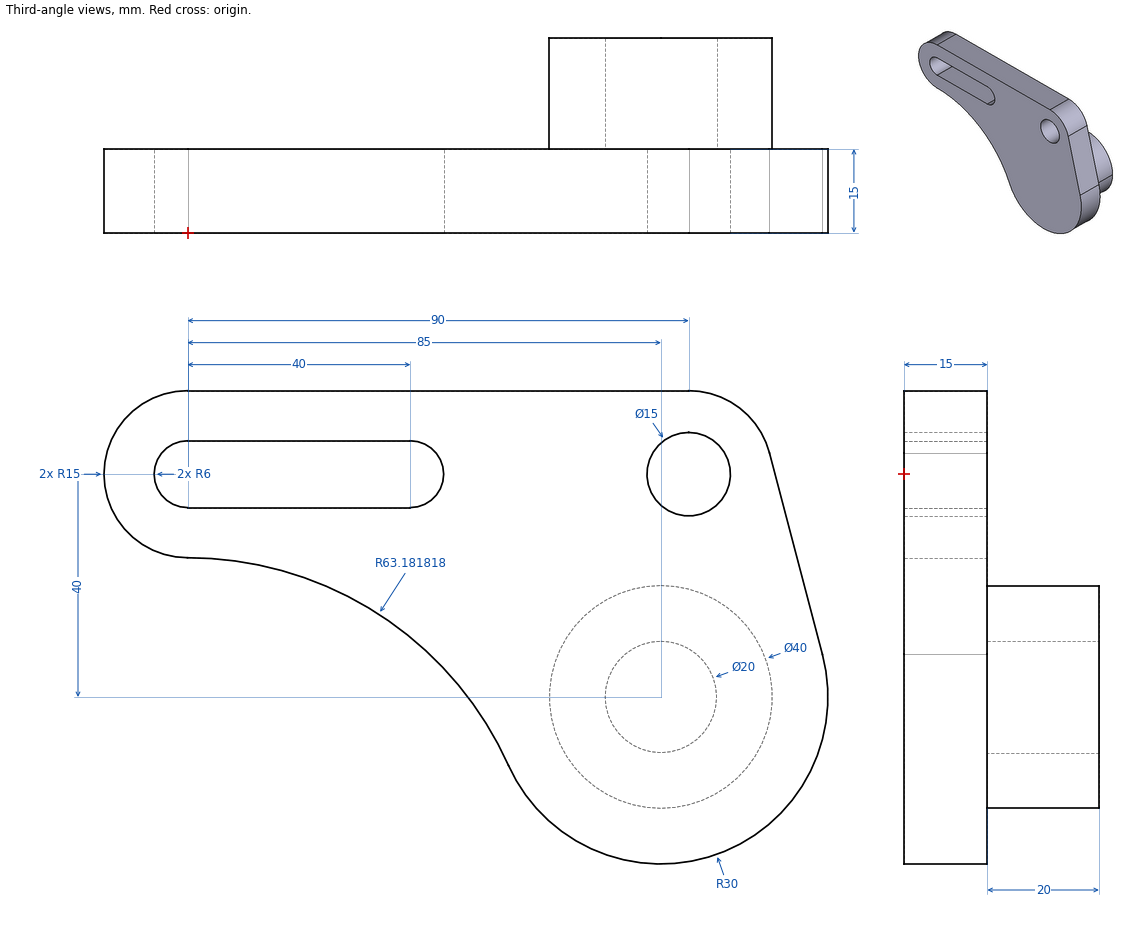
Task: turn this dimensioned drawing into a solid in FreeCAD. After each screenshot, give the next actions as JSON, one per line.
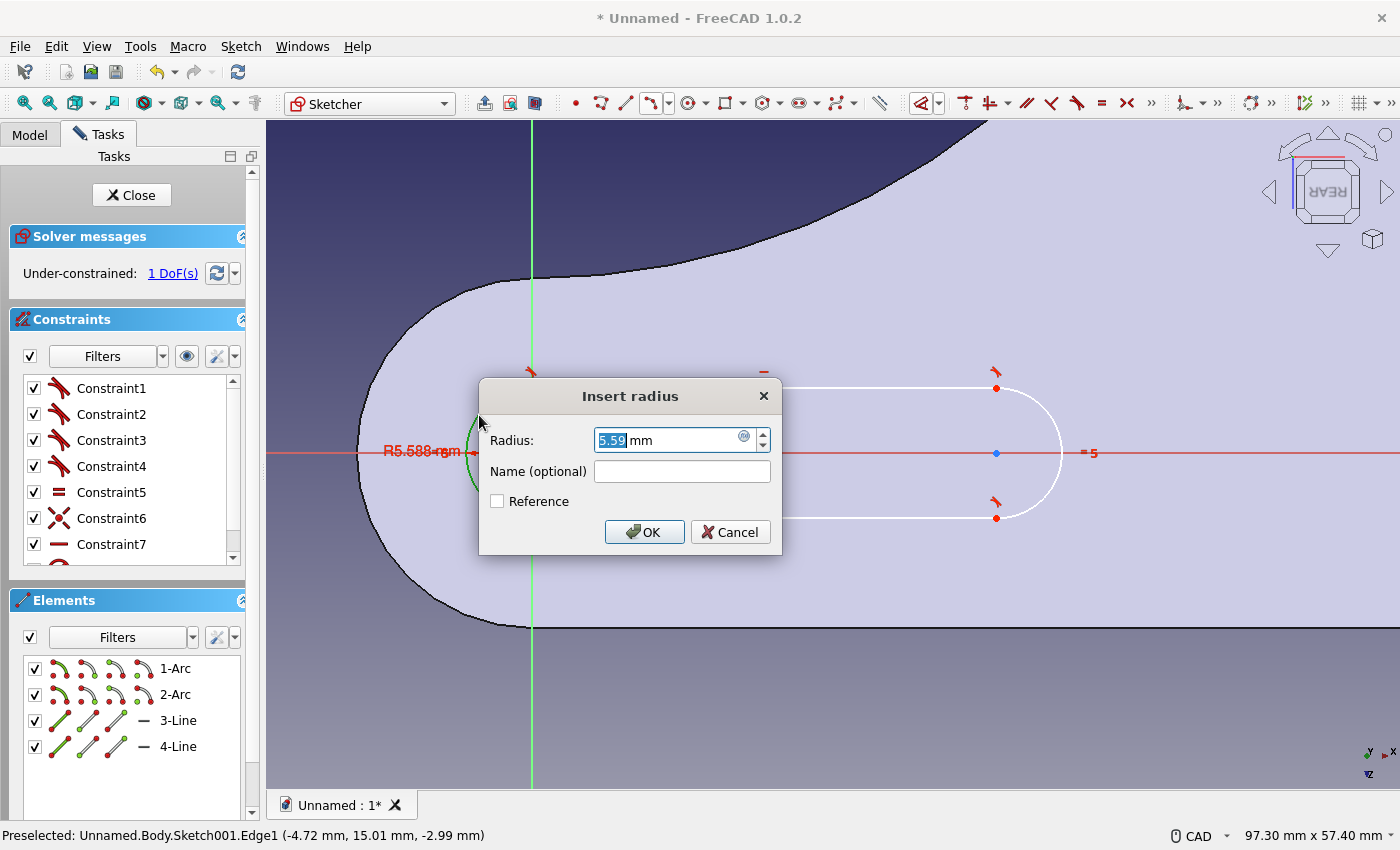
{"action": "type", "text": "6"}
{"action": "key", "text": "Return"}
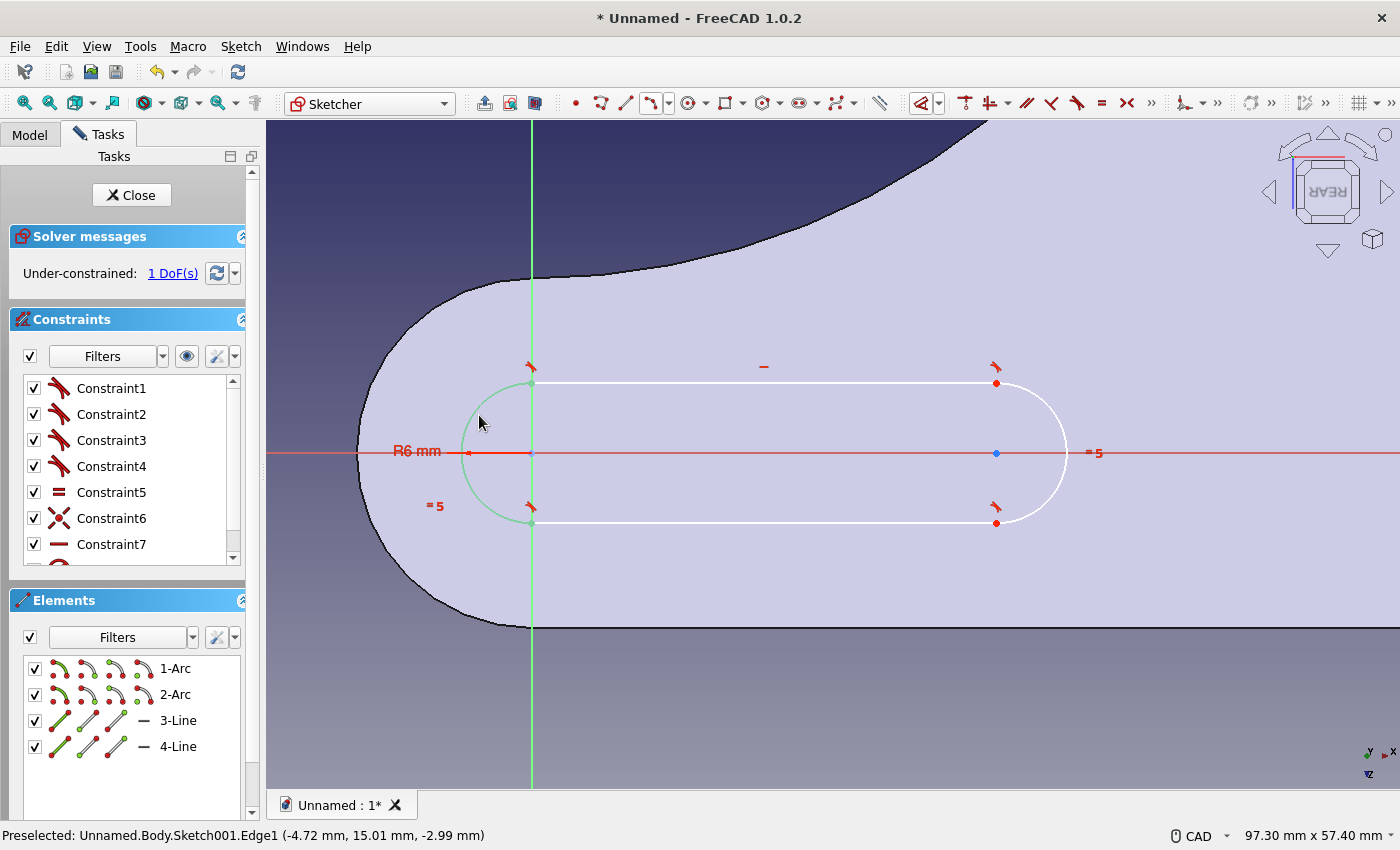
{"action": "left_click", "coordinate": [671, 383]}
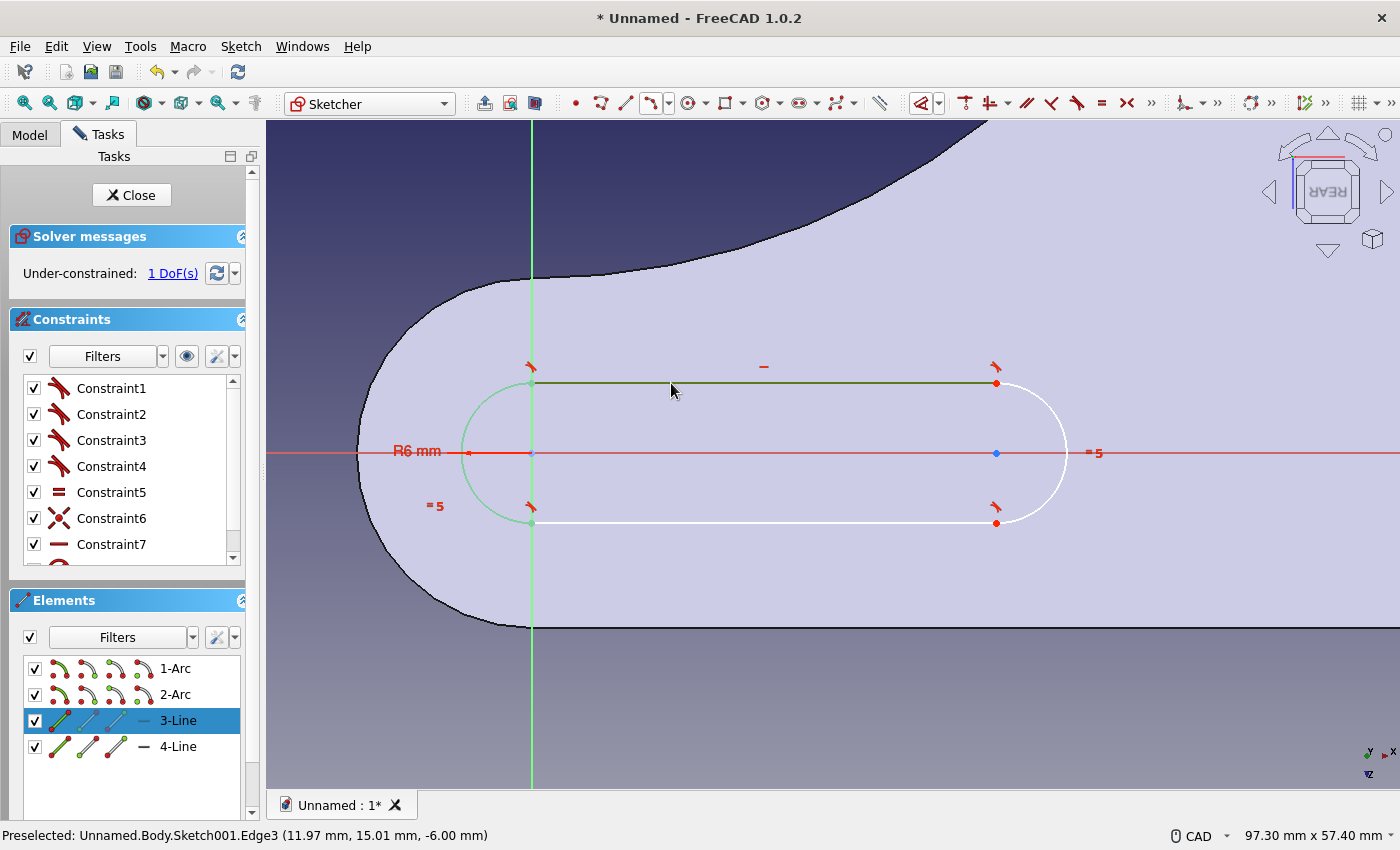
{"action": "left_click", "coordinate": [938, 104]}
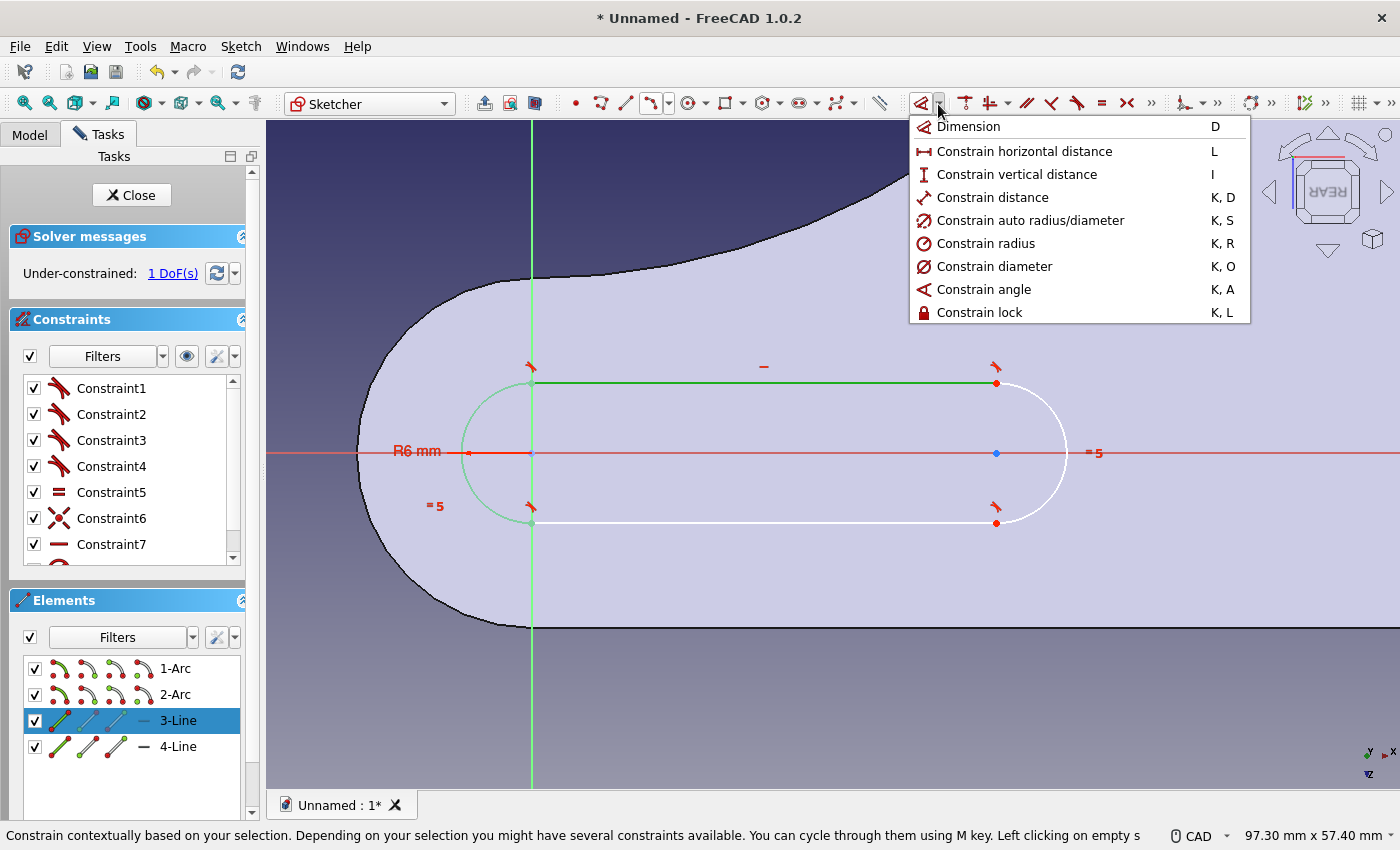
{"action": "left_click", "coordinate": [1080, 152]}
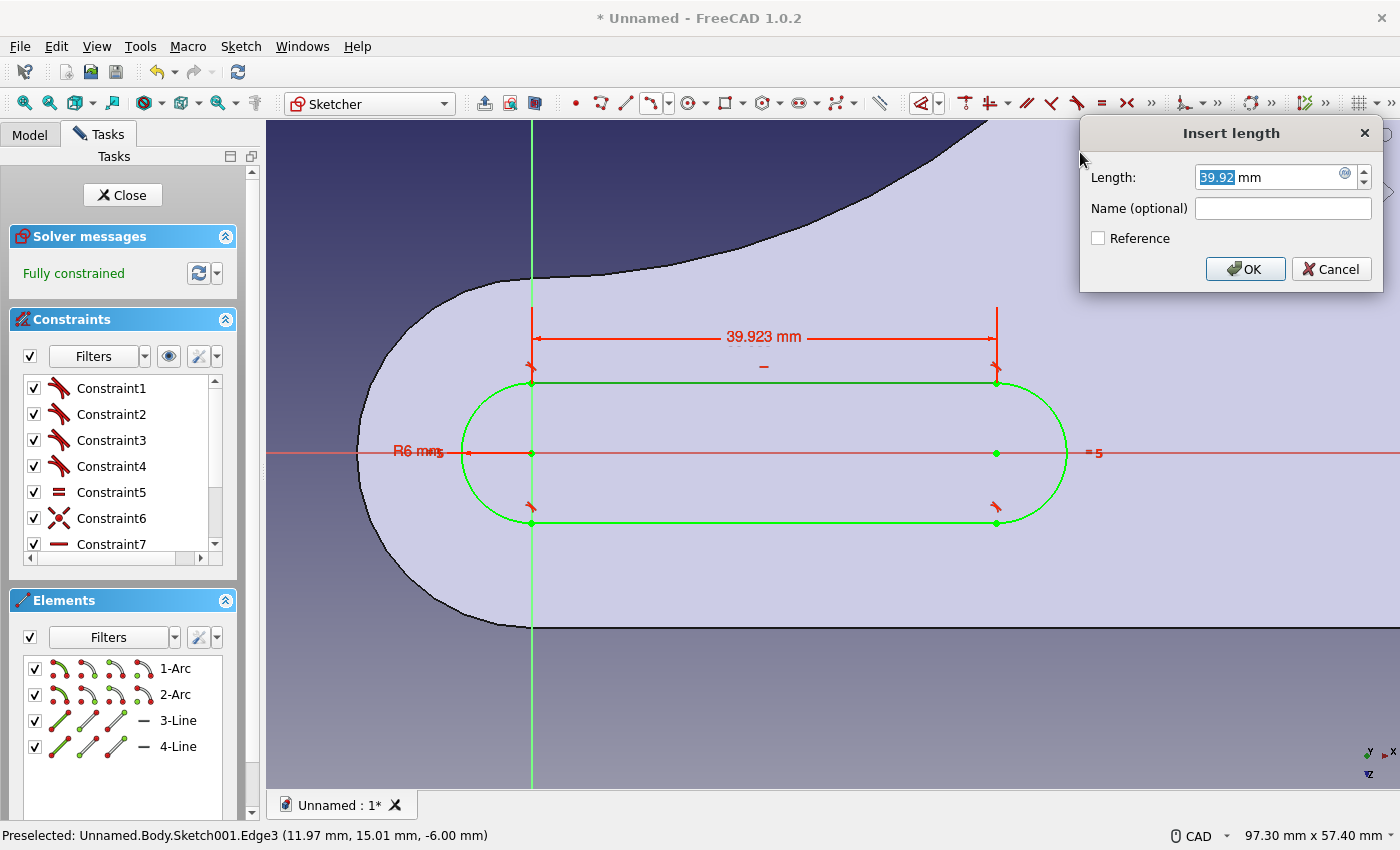
{"action": "type", "text": "40"}
{"action": "key", "text": "Return"}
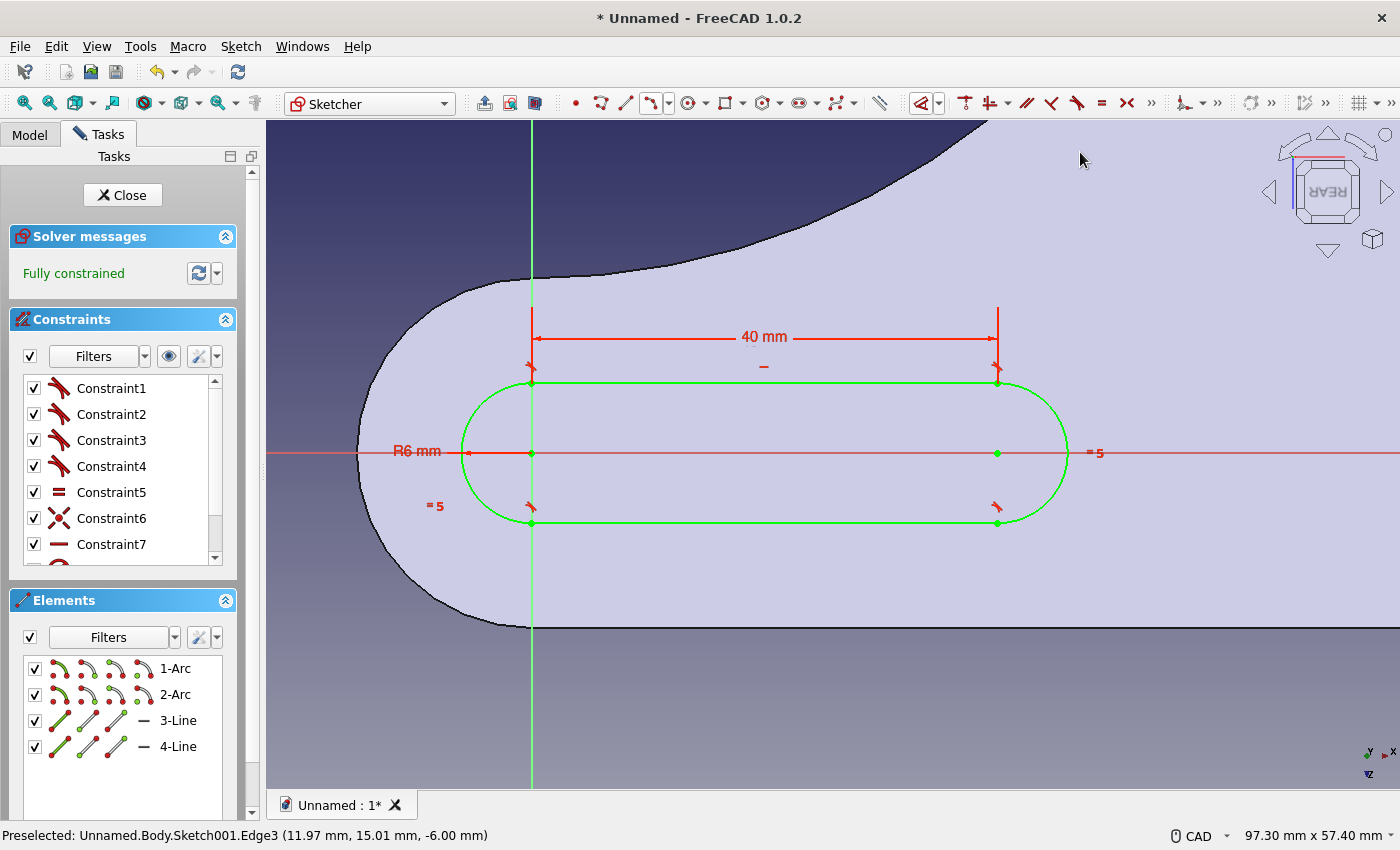
{"action": "left_click", "coordinate": [123, 195]}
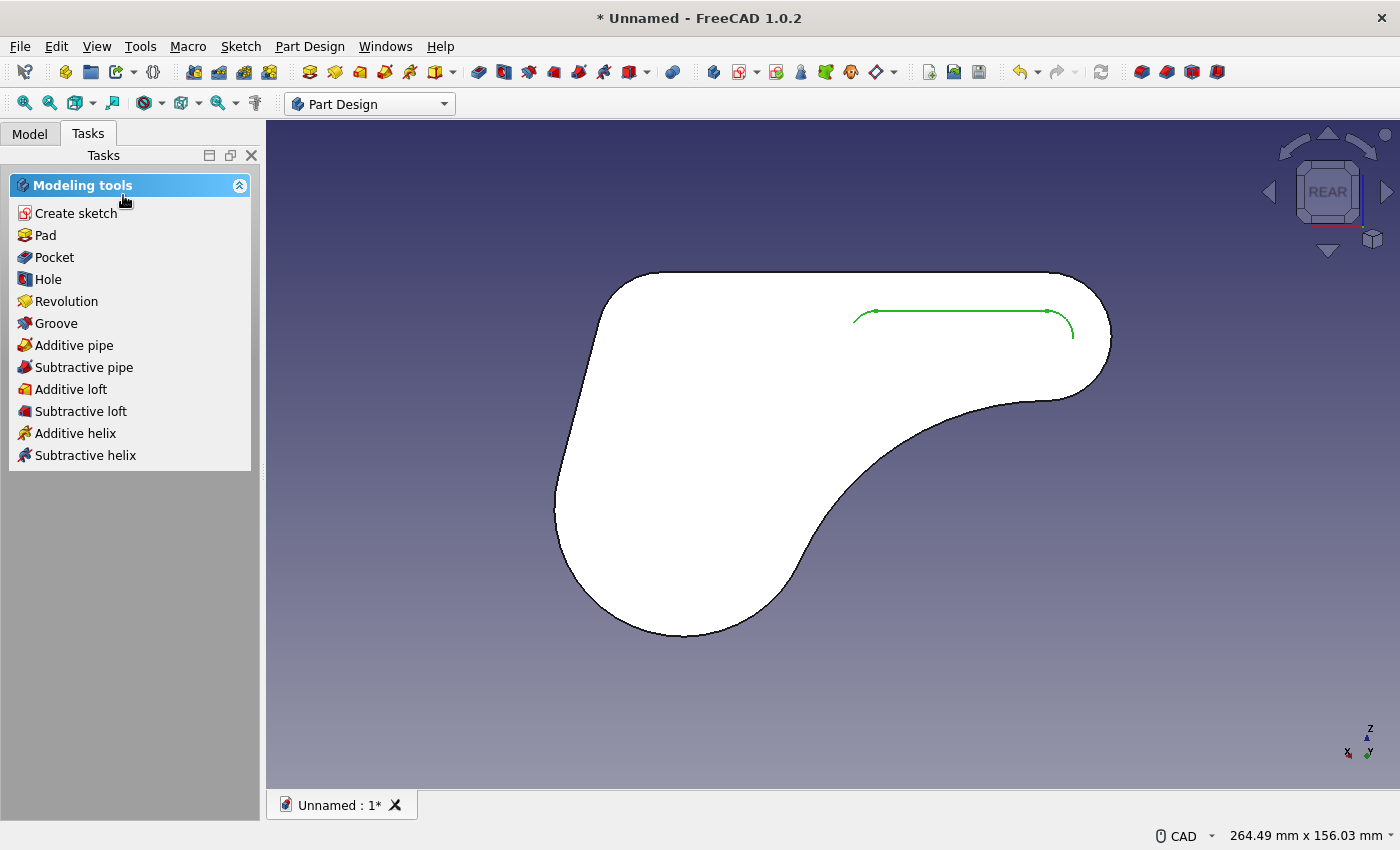
{"action": "left_click", "coordinate": [479, 72]}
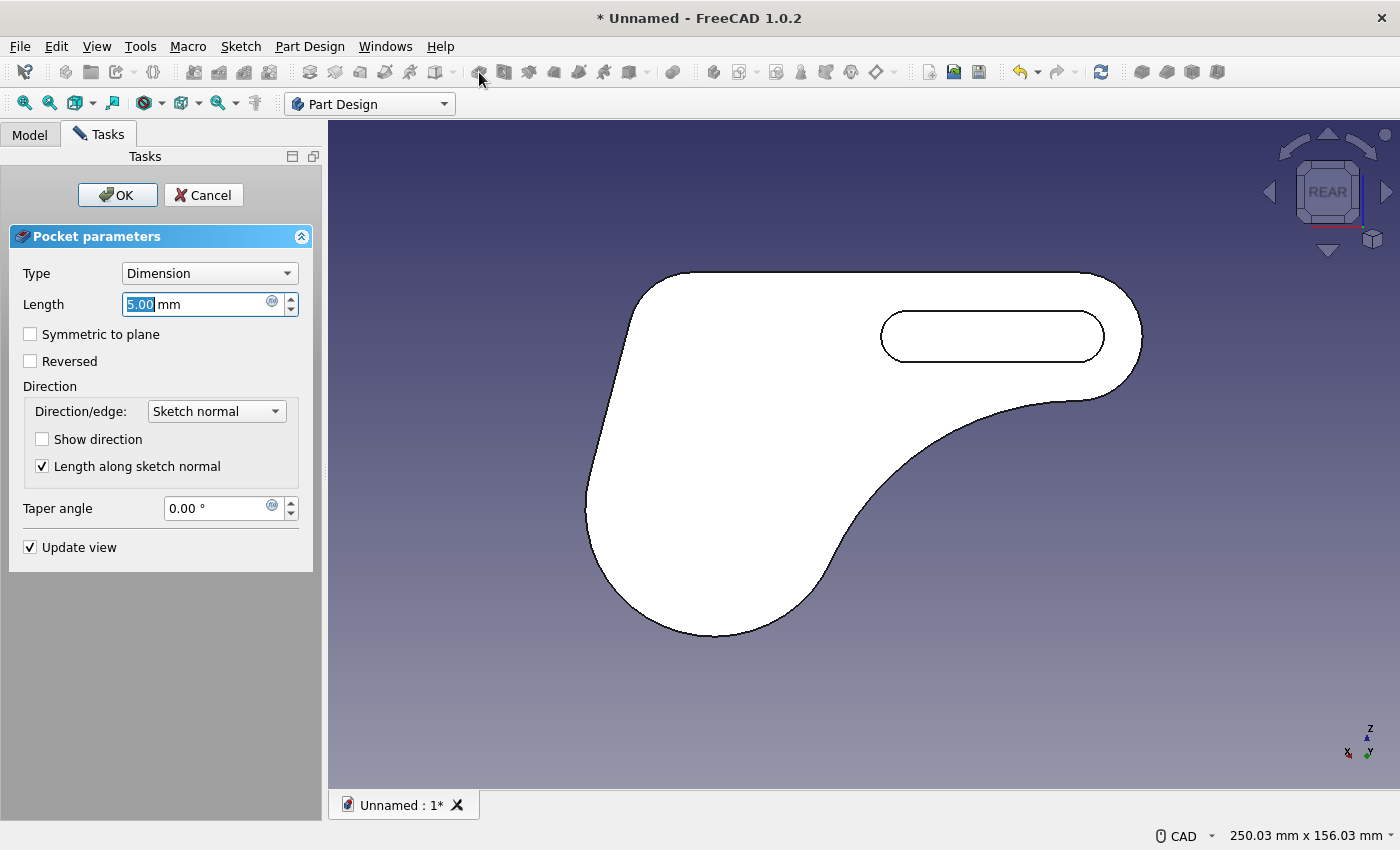
{"action": "left_click", "coordinate": [210, 274]}